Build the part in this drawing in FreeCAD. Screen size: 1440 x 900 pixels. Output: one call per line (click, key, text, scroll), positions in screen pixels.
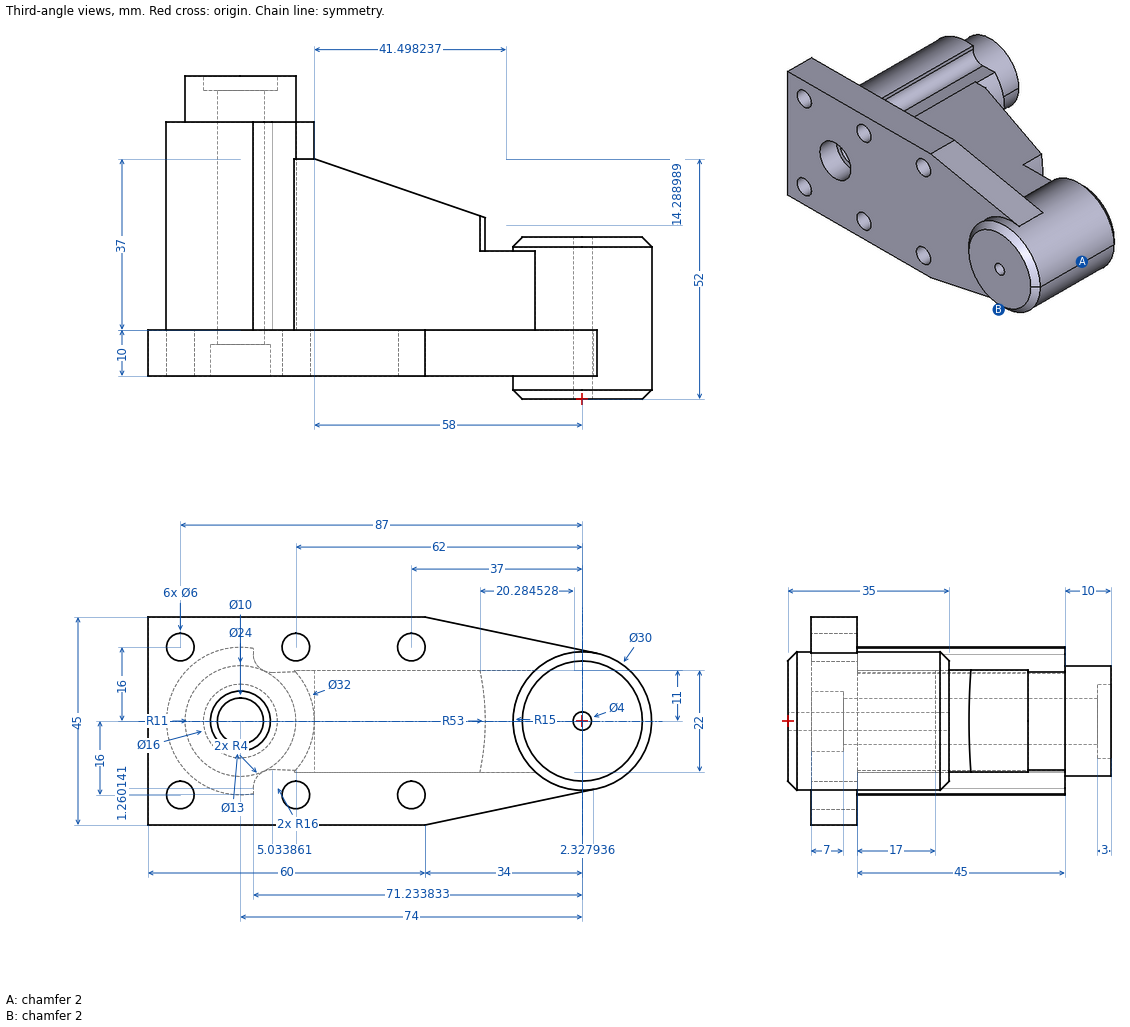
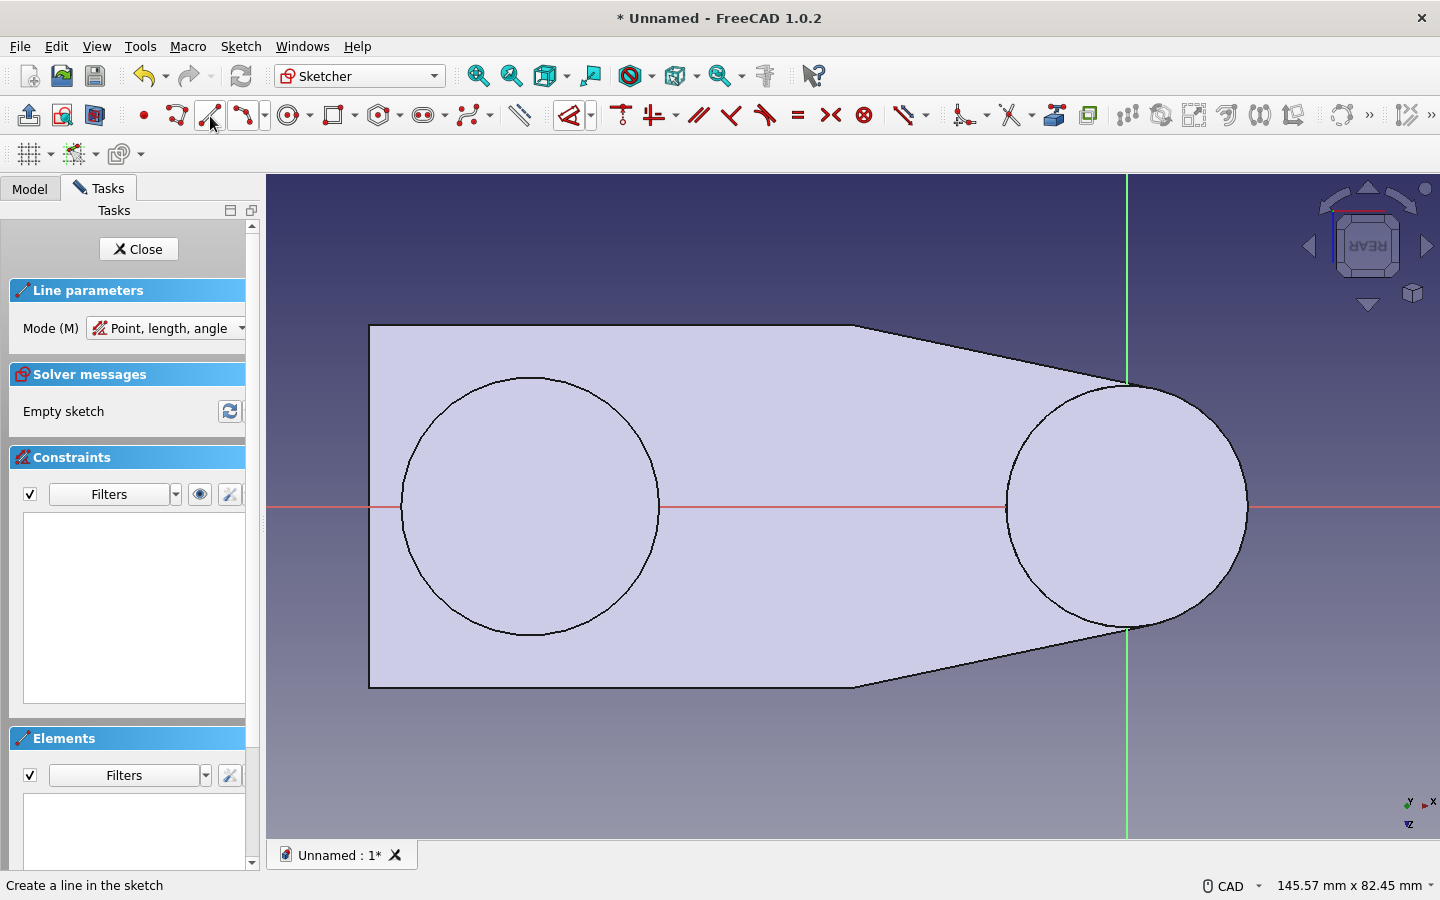
click(948, 418)
click(530, 418)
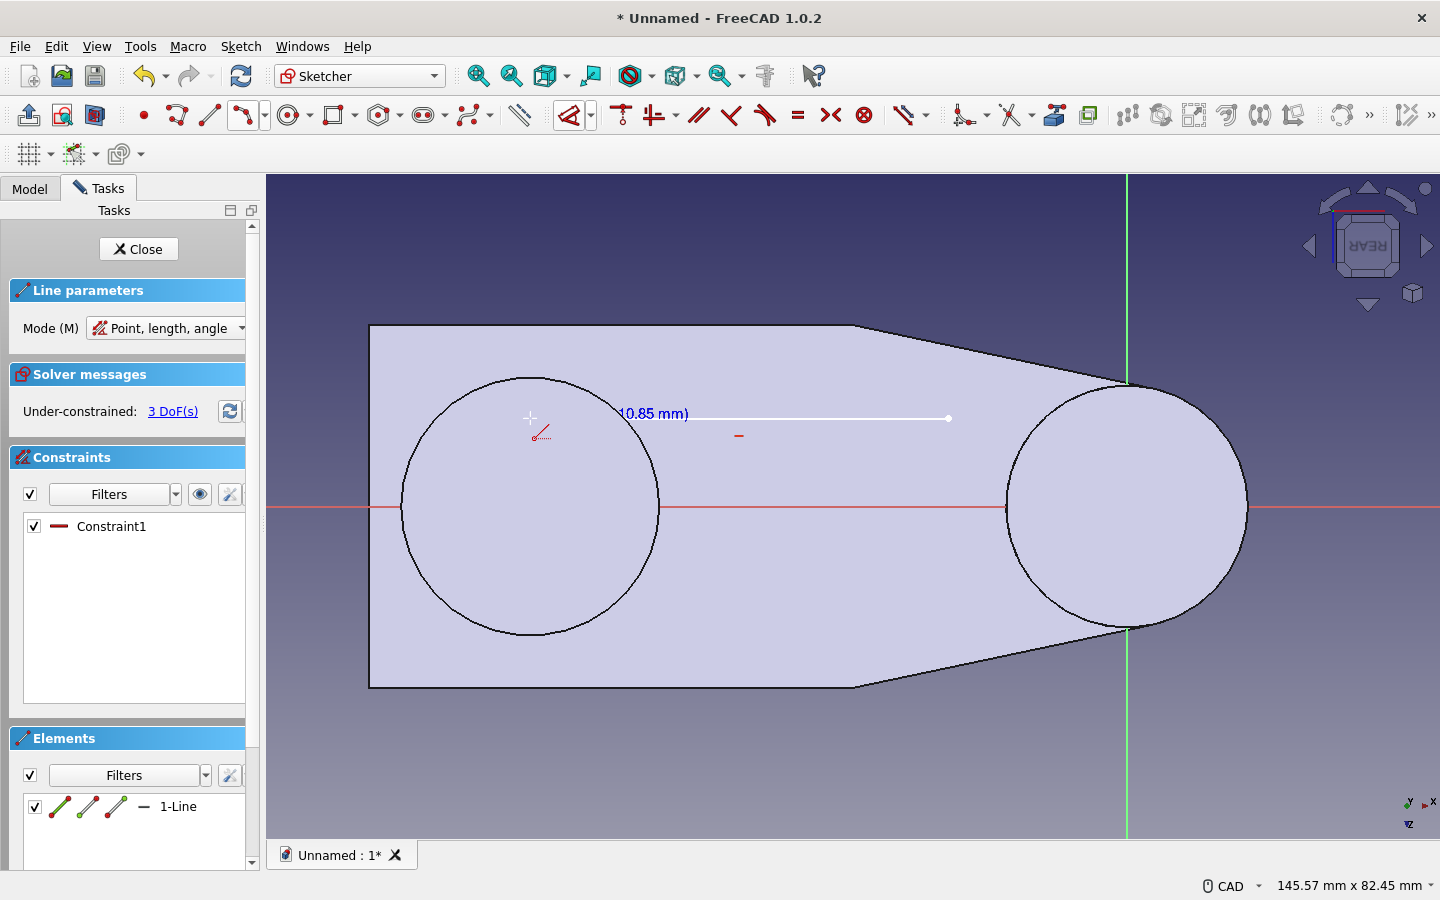
click(530, 595)
click(948, 595)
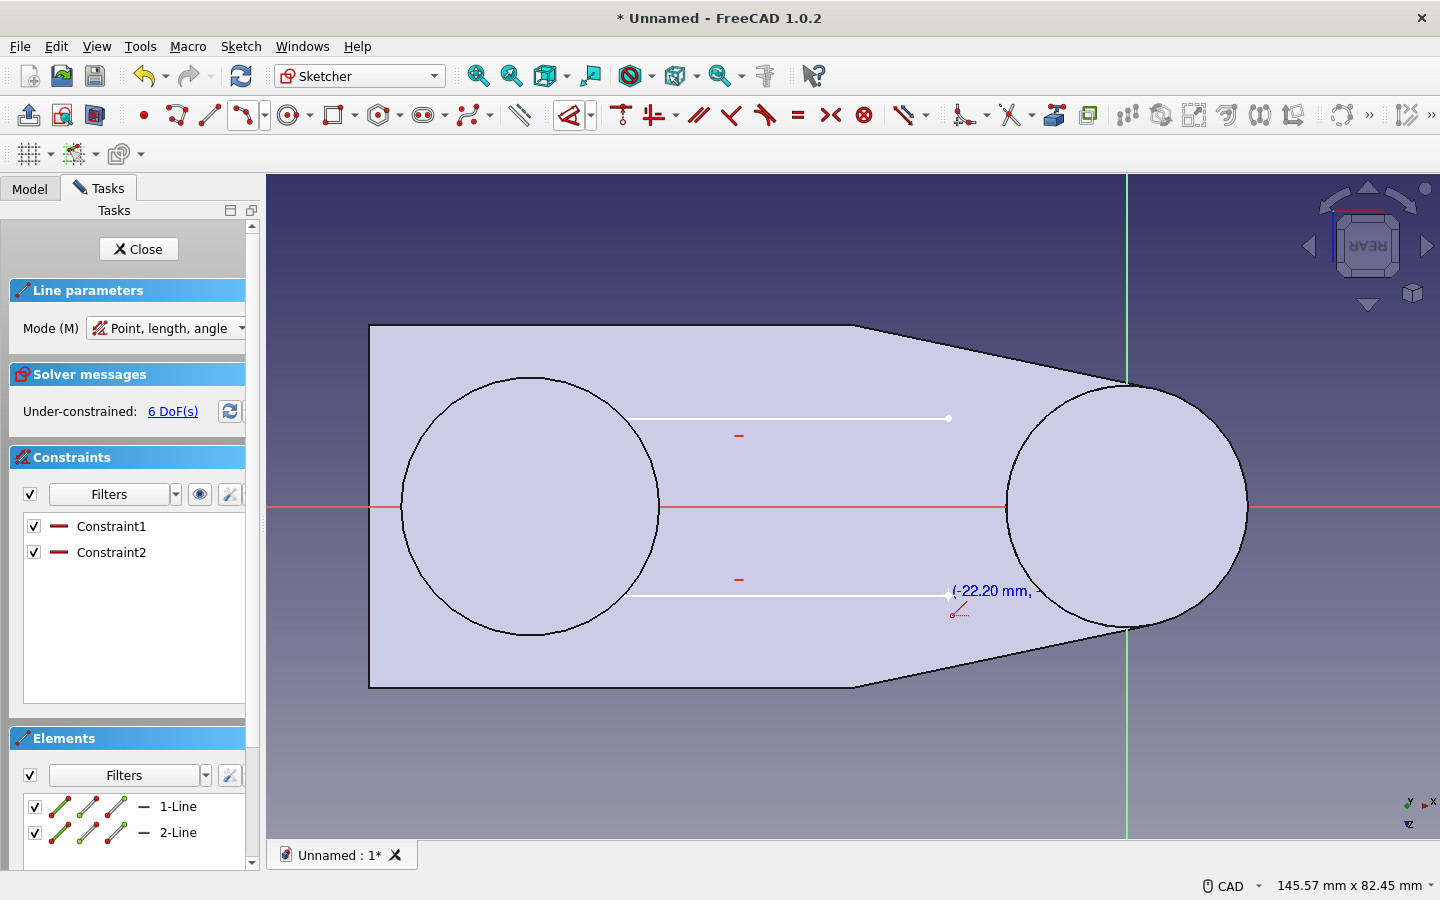
click(242, 116)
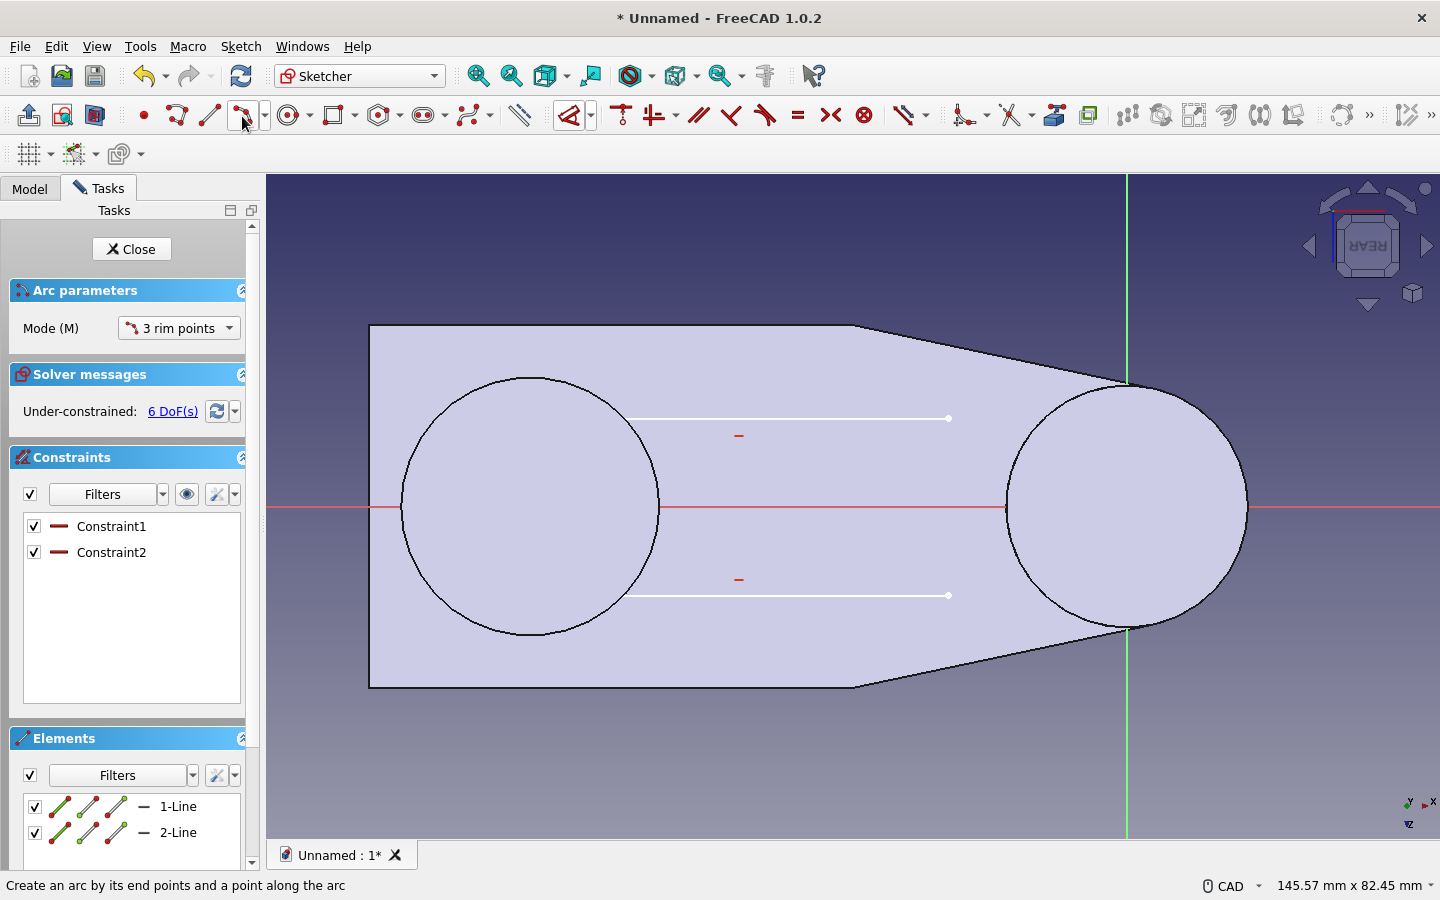
click(530, 419)
click(530, 596)
click(446, 479)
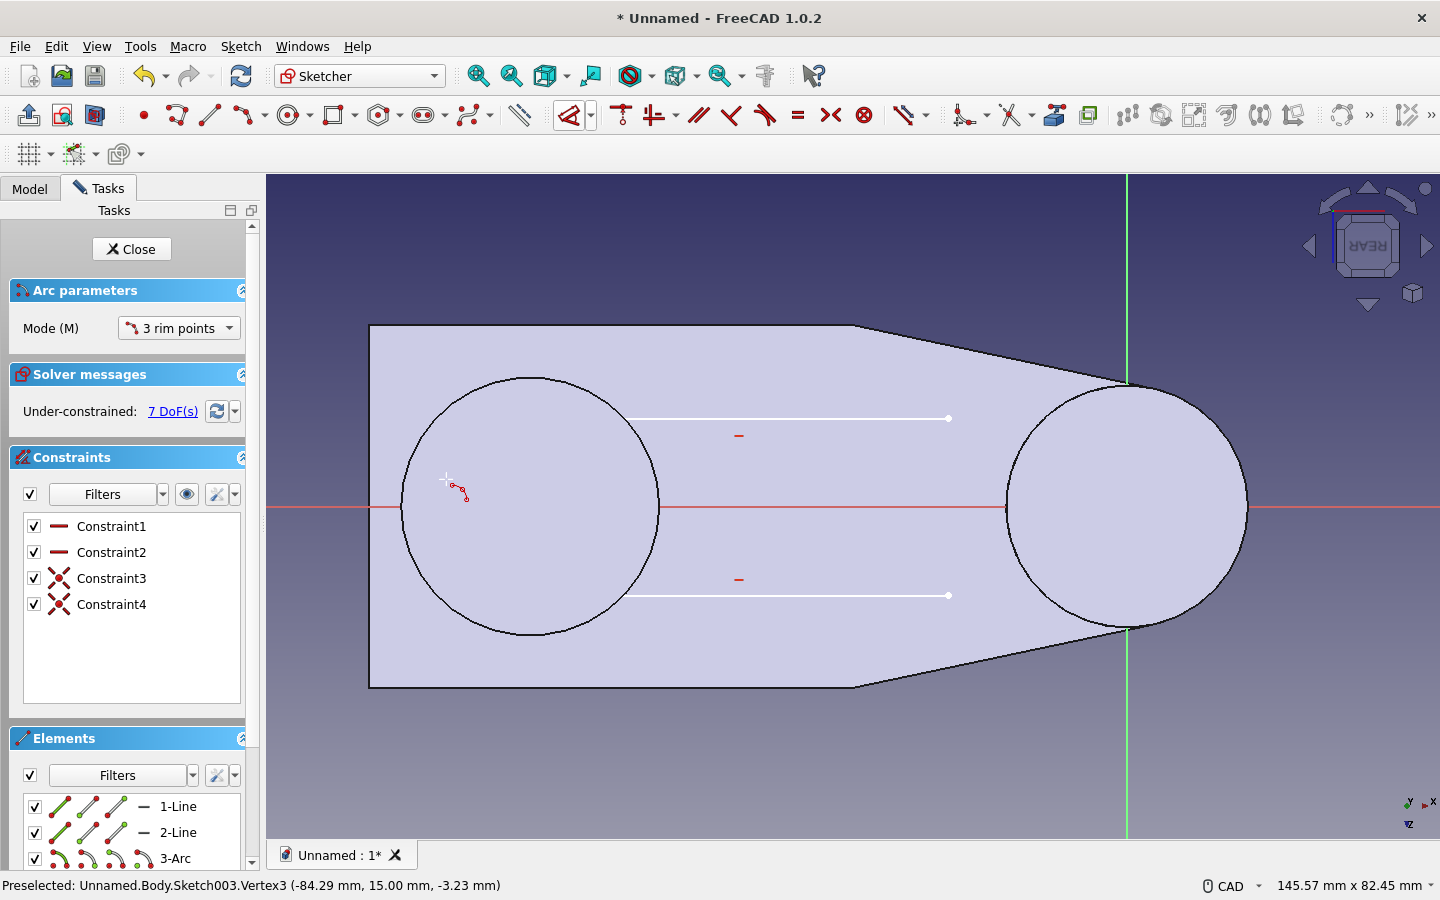
click(948, 596)
click(948, 419)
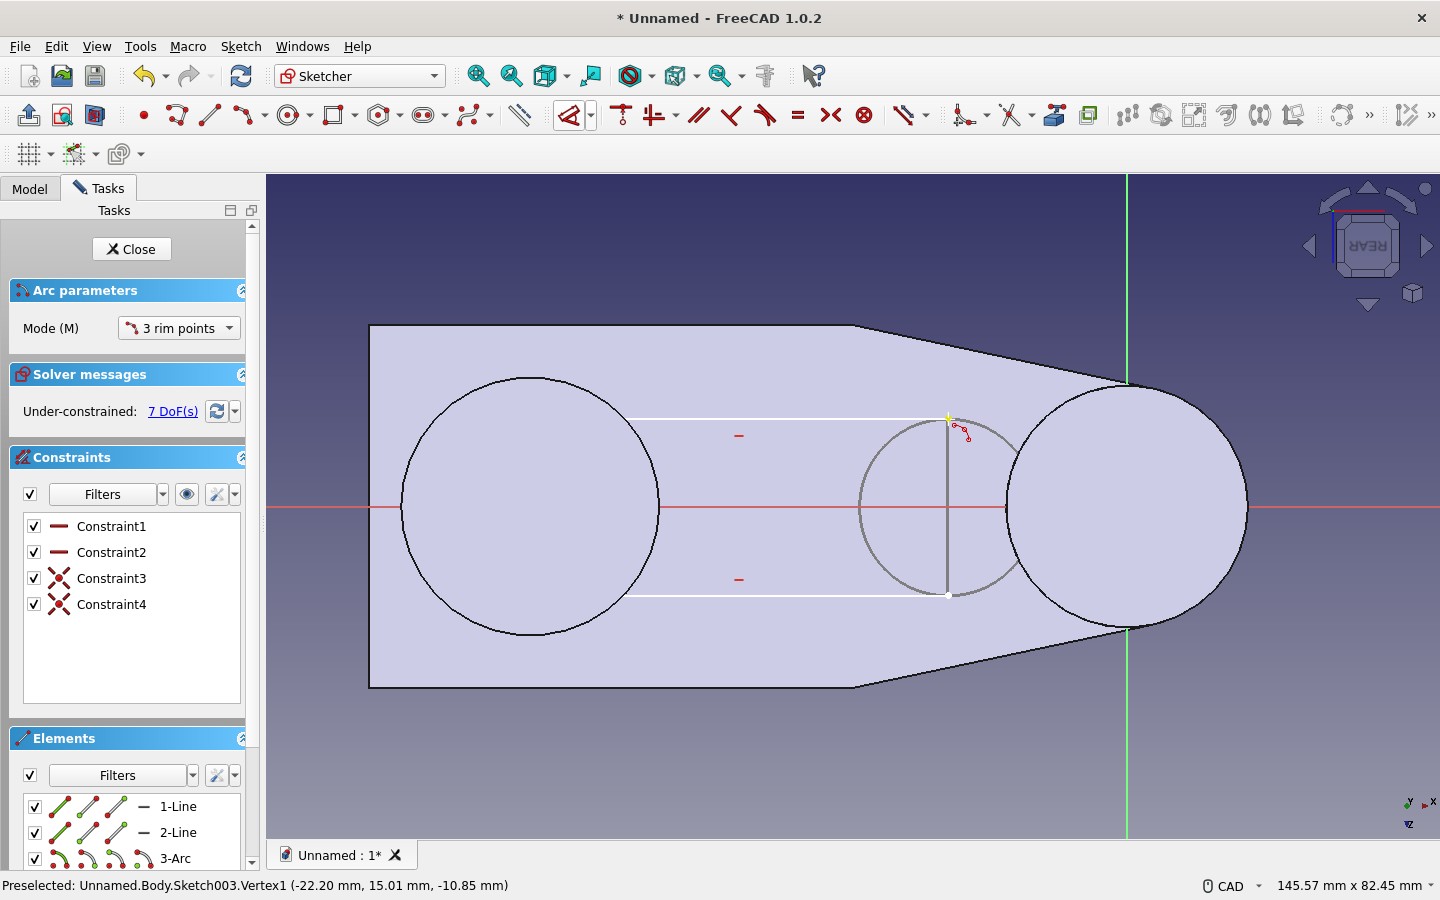
scroll(957, 524, up, 3)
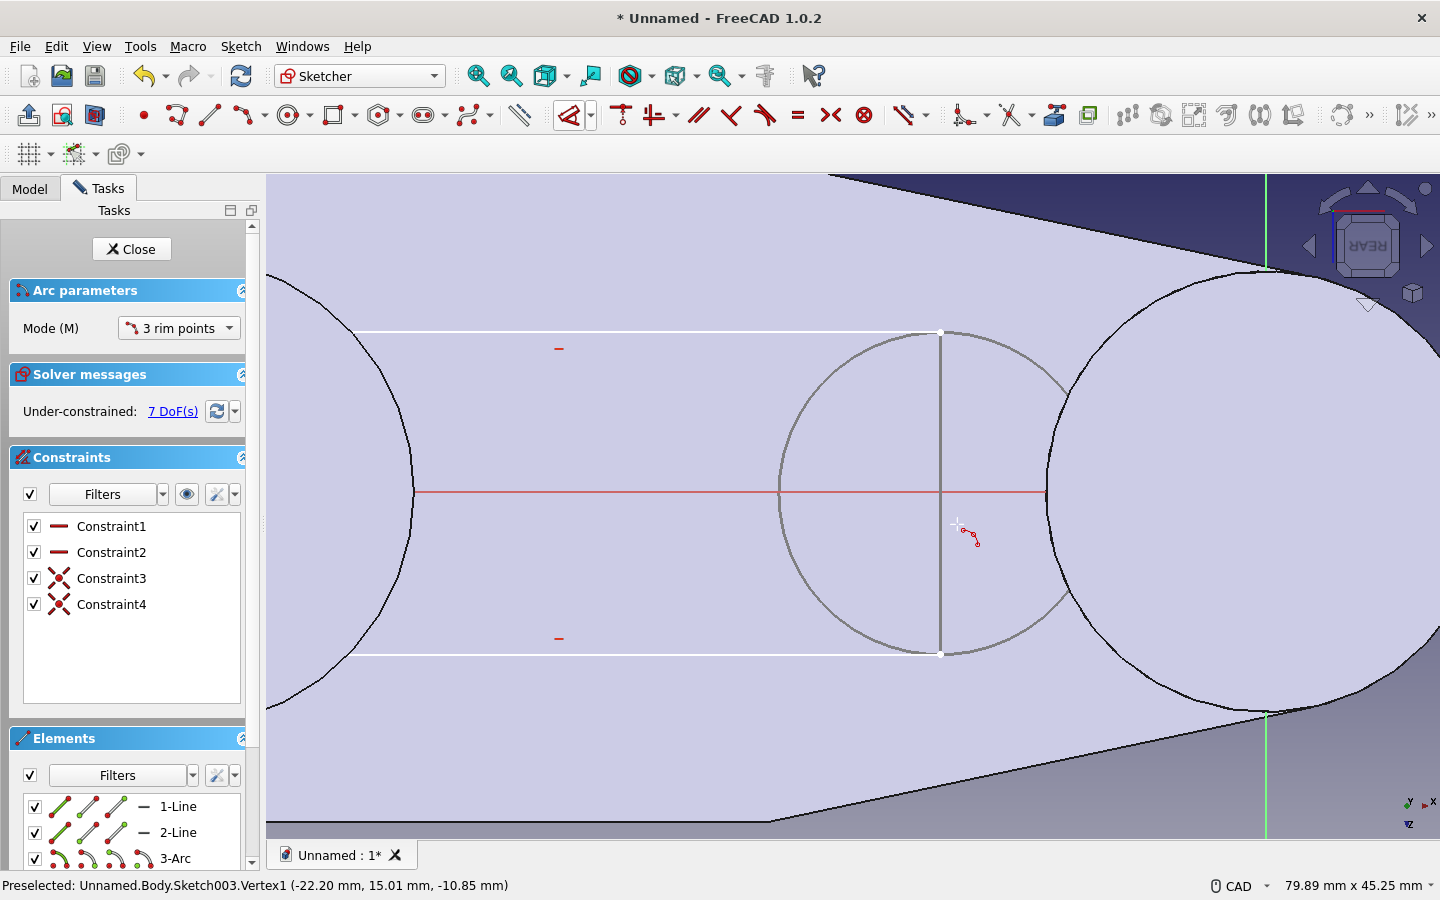
click(957, 524)
key(Escape)